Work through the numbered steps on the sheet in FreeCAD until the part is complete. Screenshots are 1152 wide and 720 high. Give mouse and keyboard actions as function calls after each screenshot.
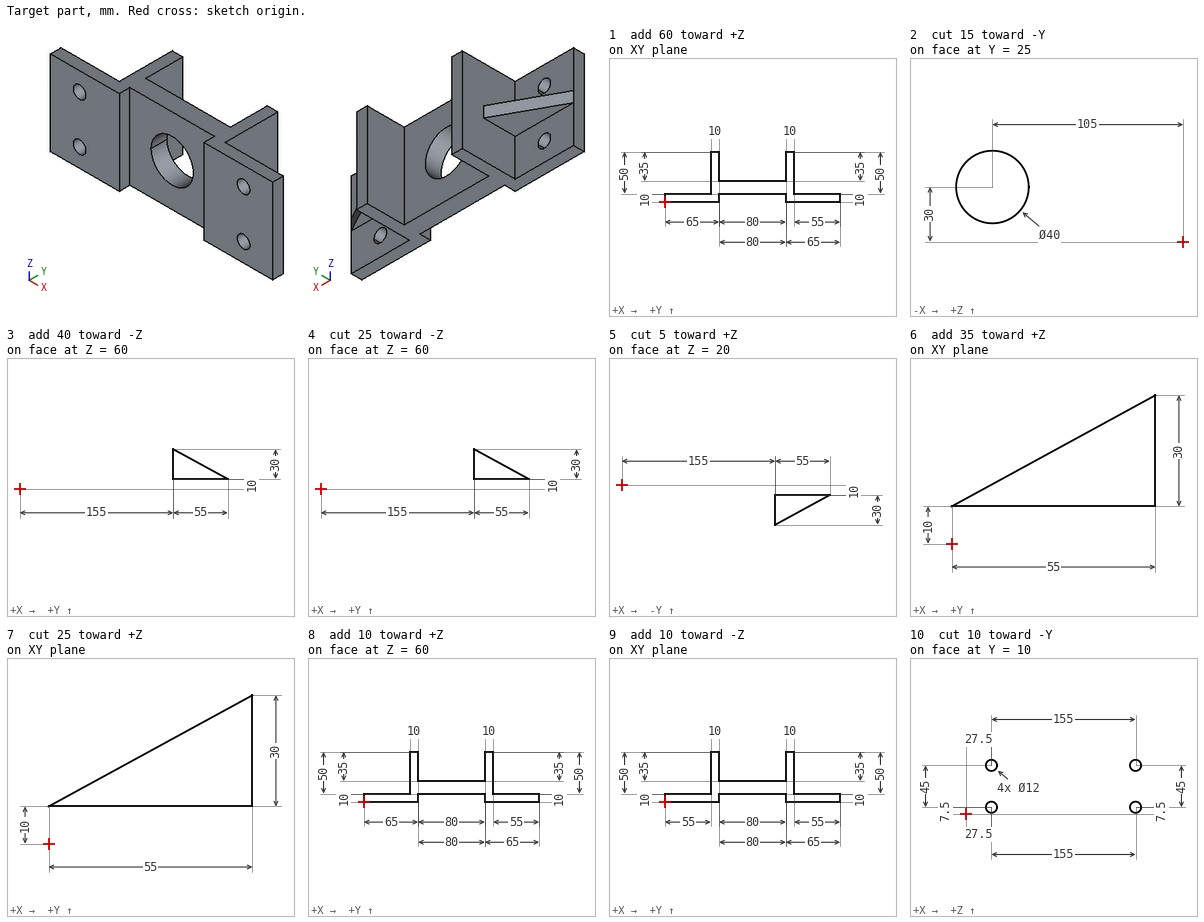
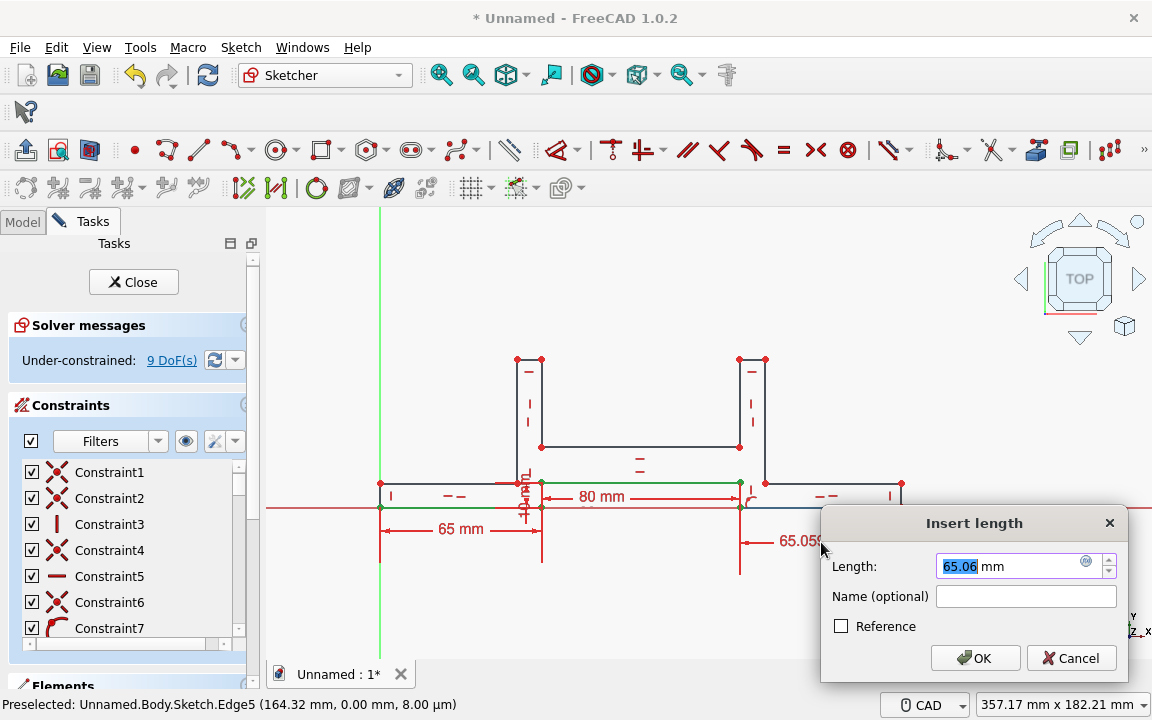
text(65)
key(Return)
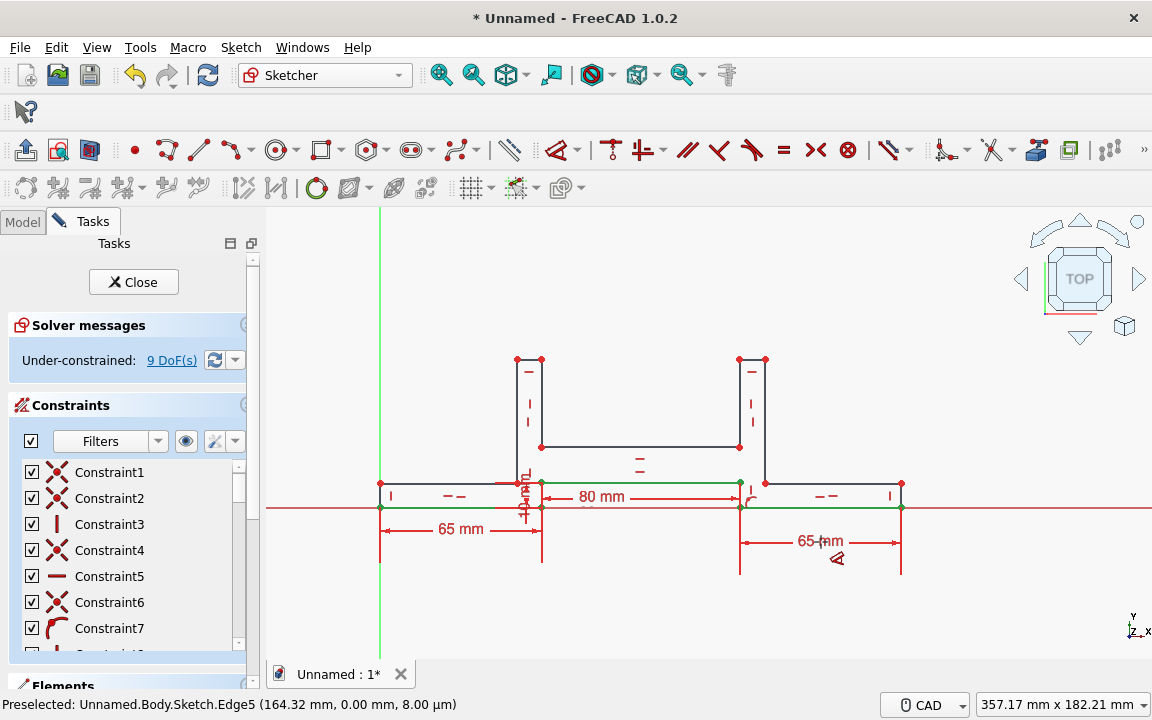
scroll(901, 498, up, 3)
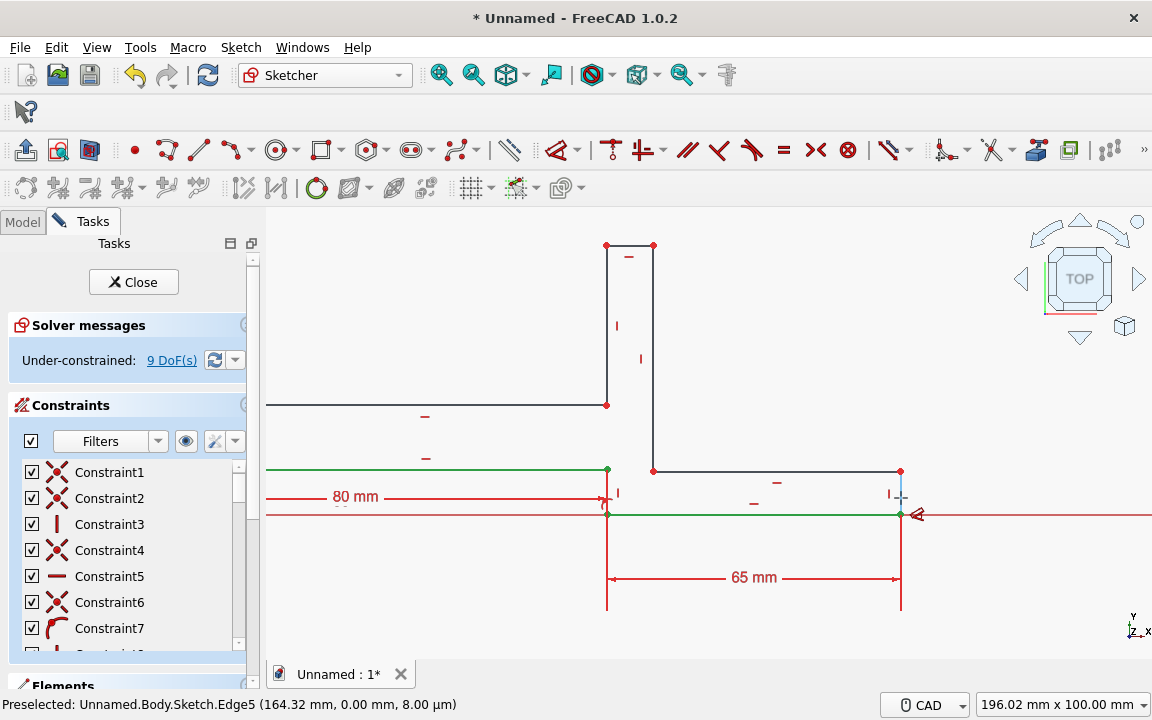
click(901, 498)
click(935, 493)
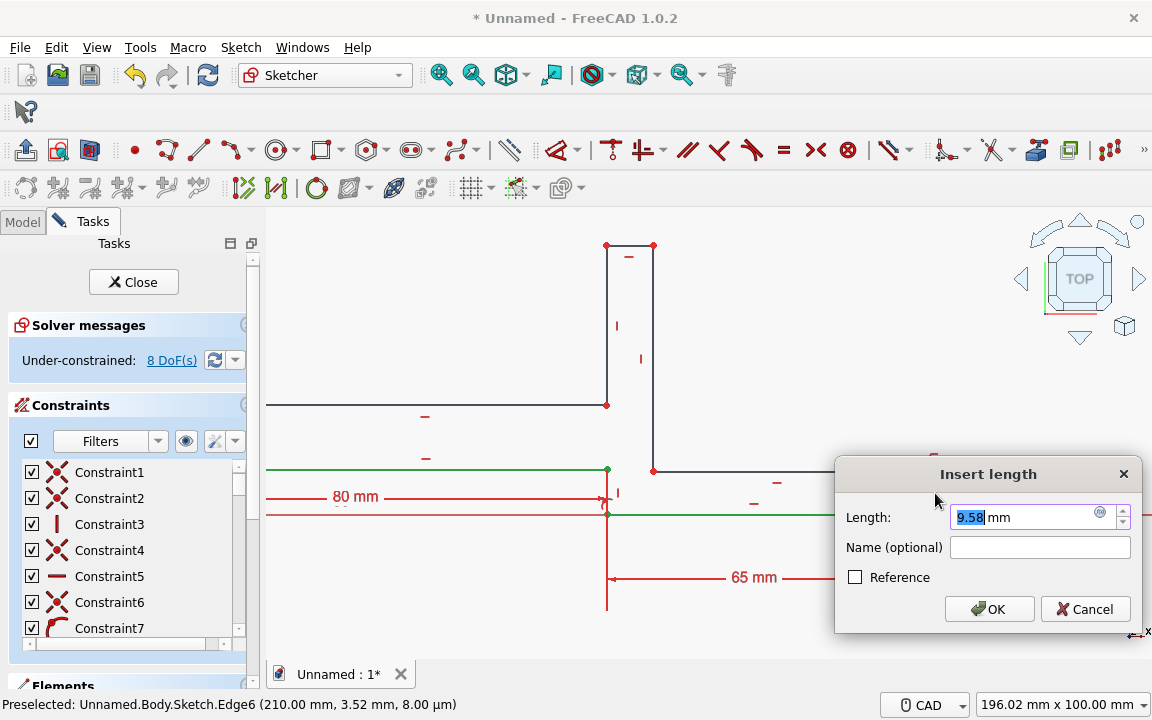
text(10)
key(Return)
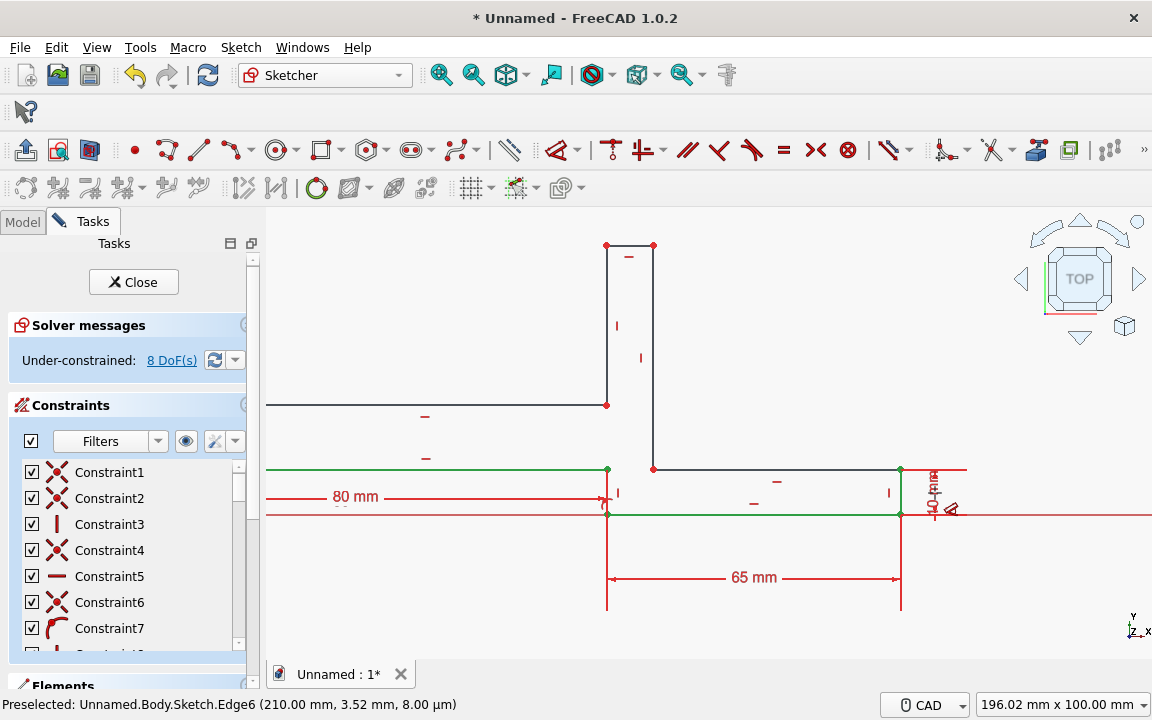
click(827, 470)
click(777, 436)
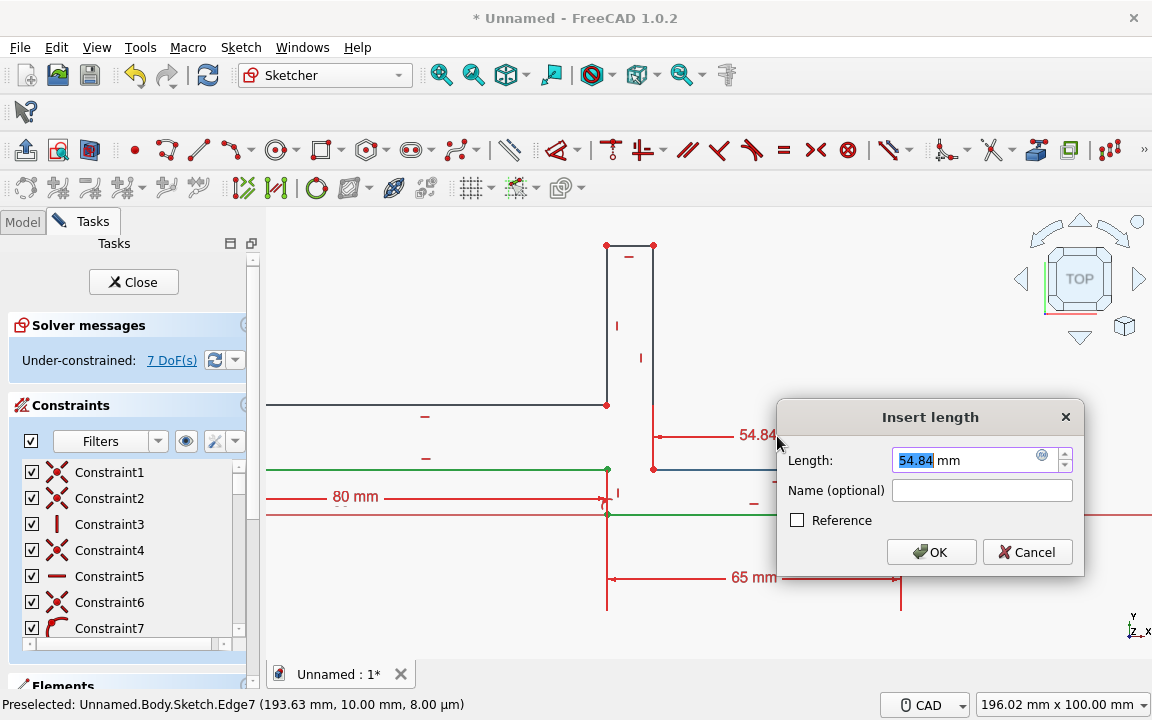
text(55)
key(Return)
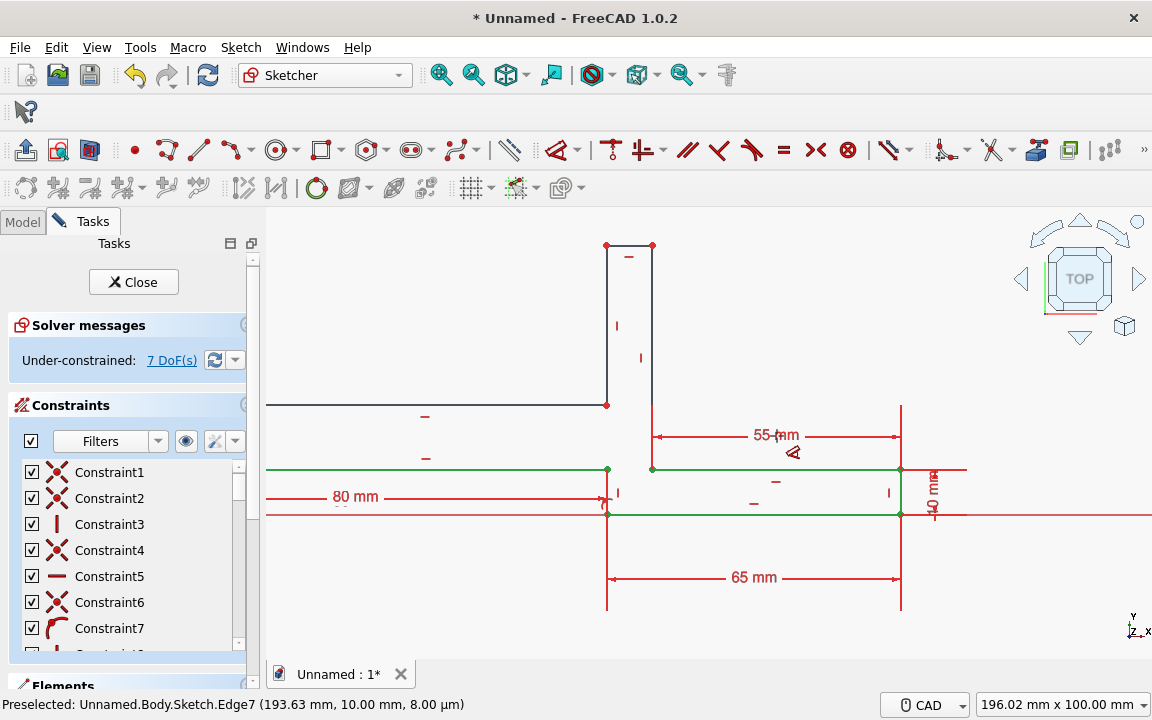
click(652, 402)
click(686, 358)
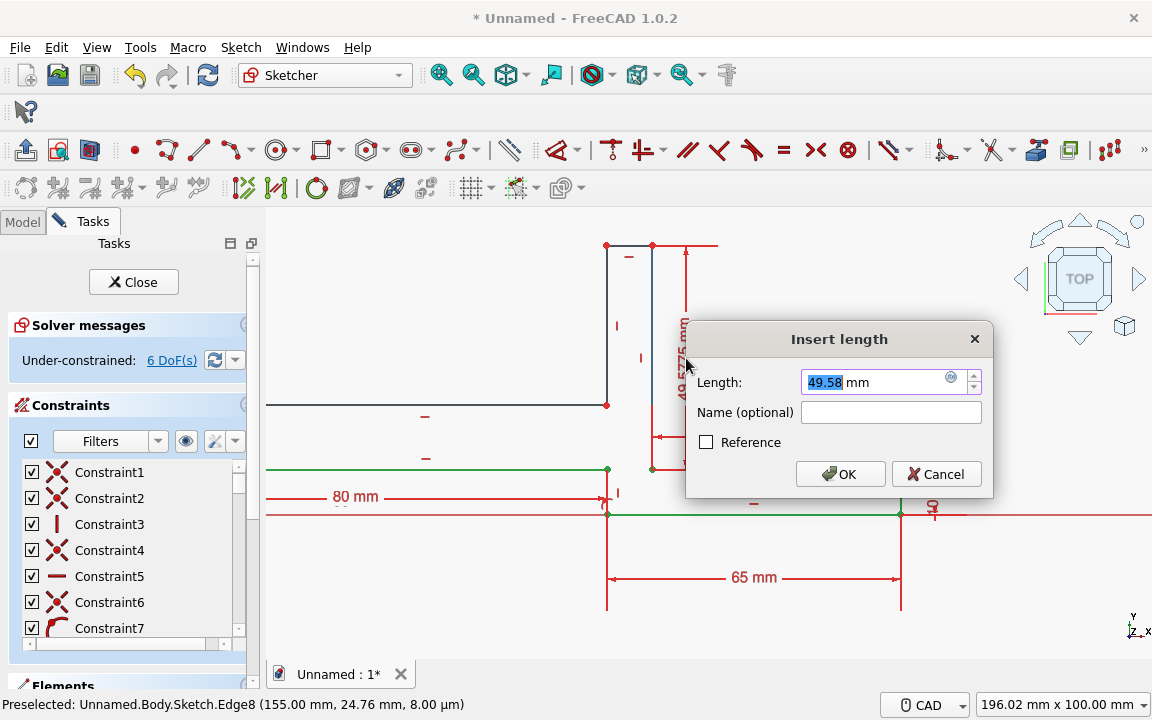
text(50)
key(Return)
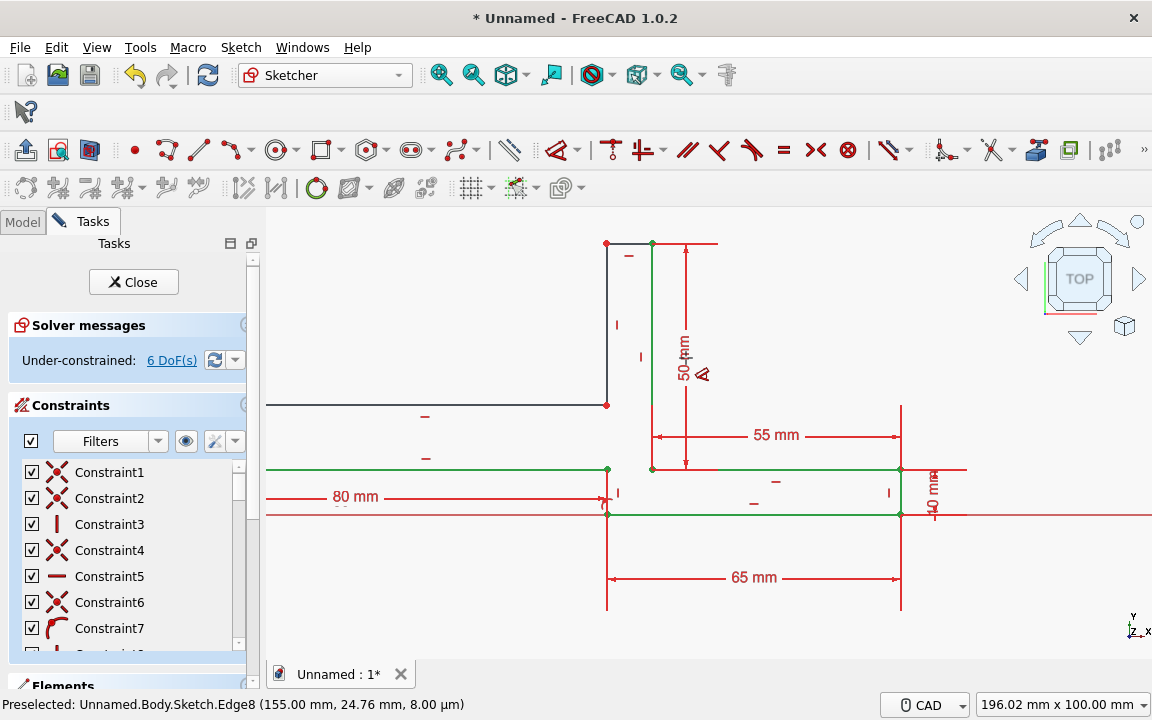
click(639, 244)
click(629, 278)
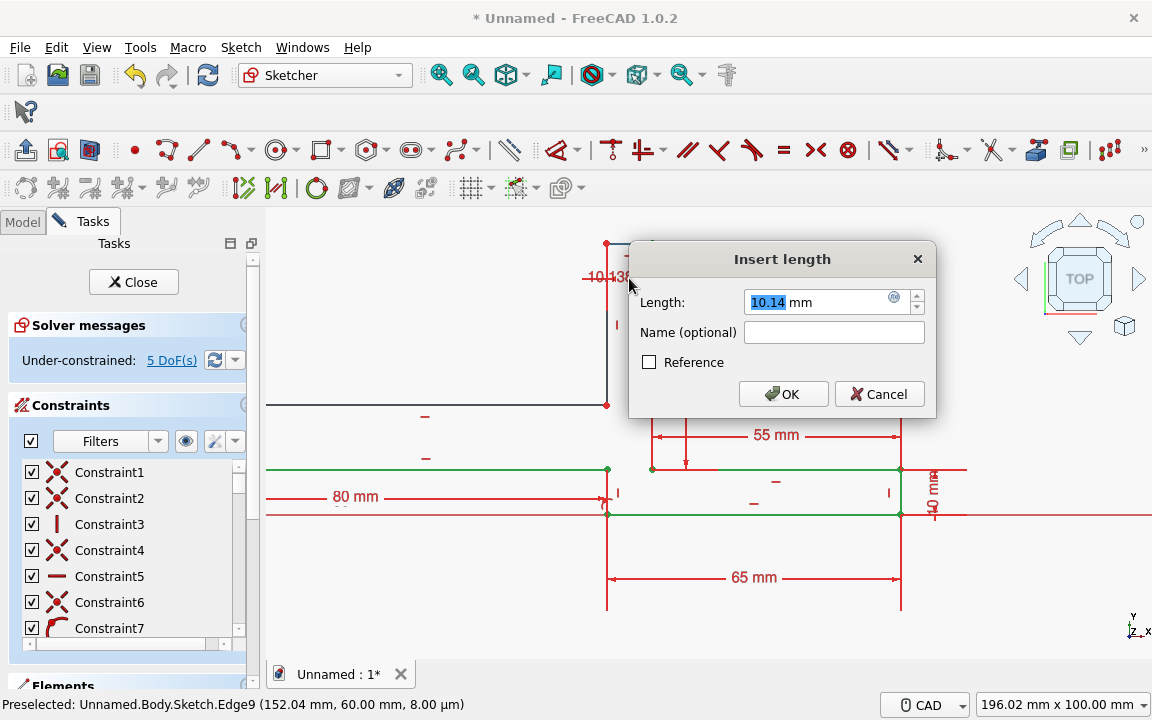
text(10)
key(Return)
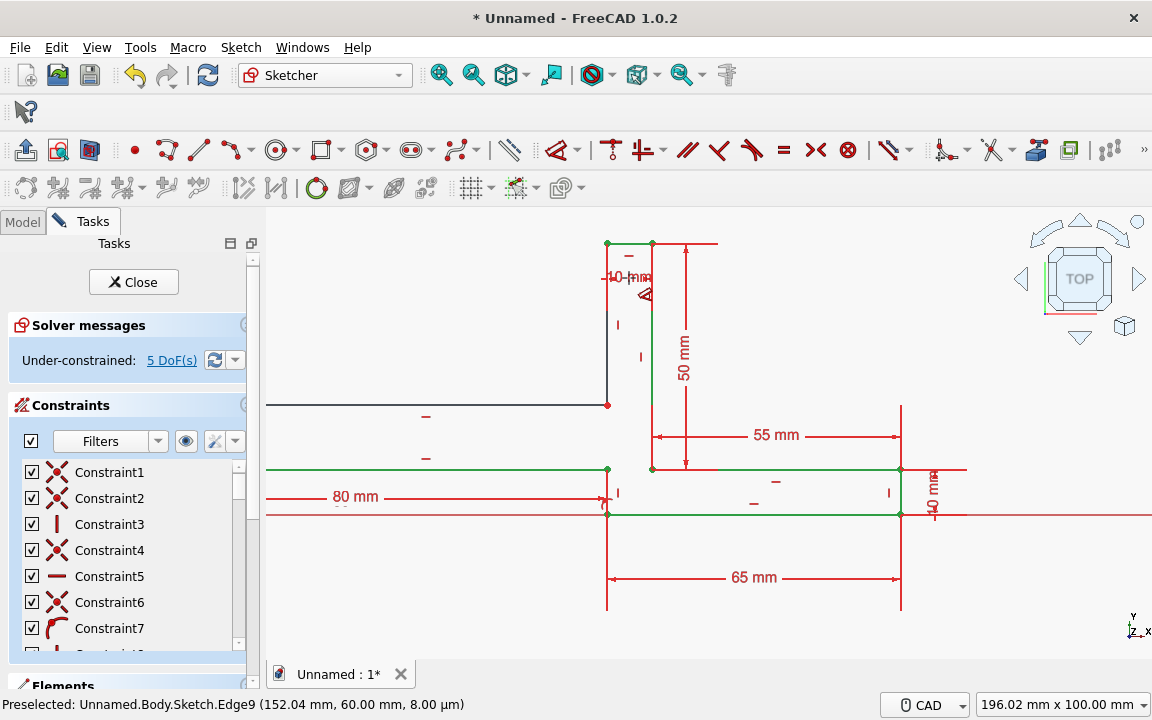
click(607, 292)
click(573, 324)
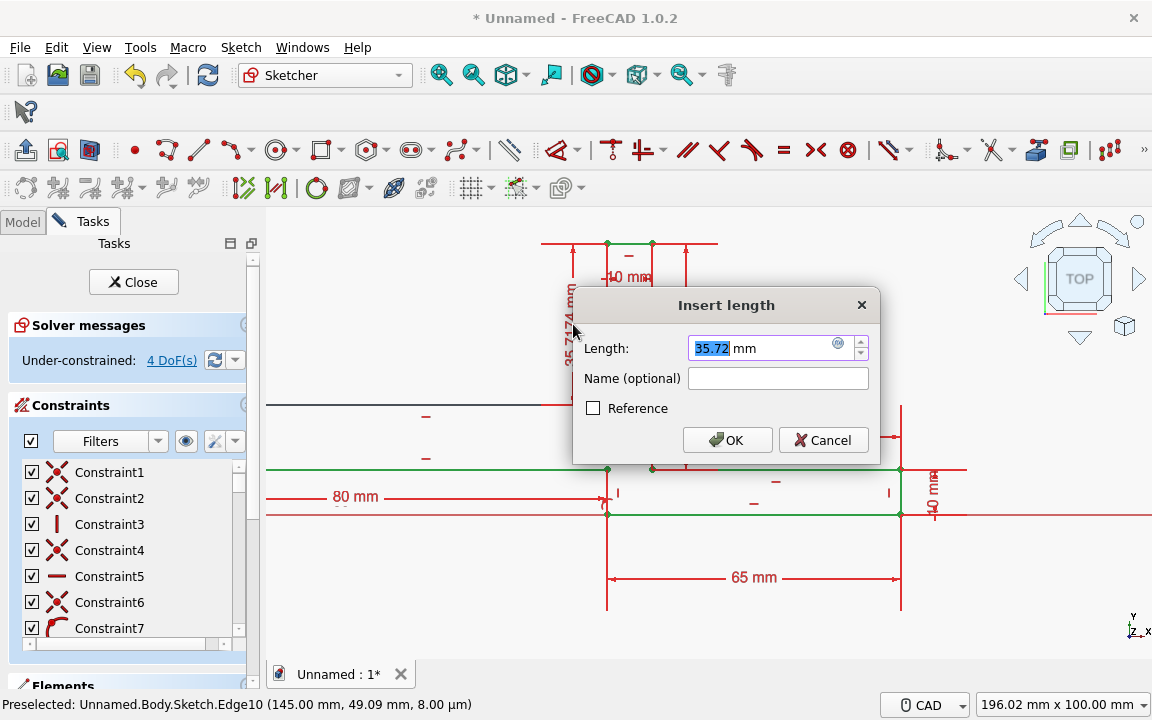
text(35)
key(Return)